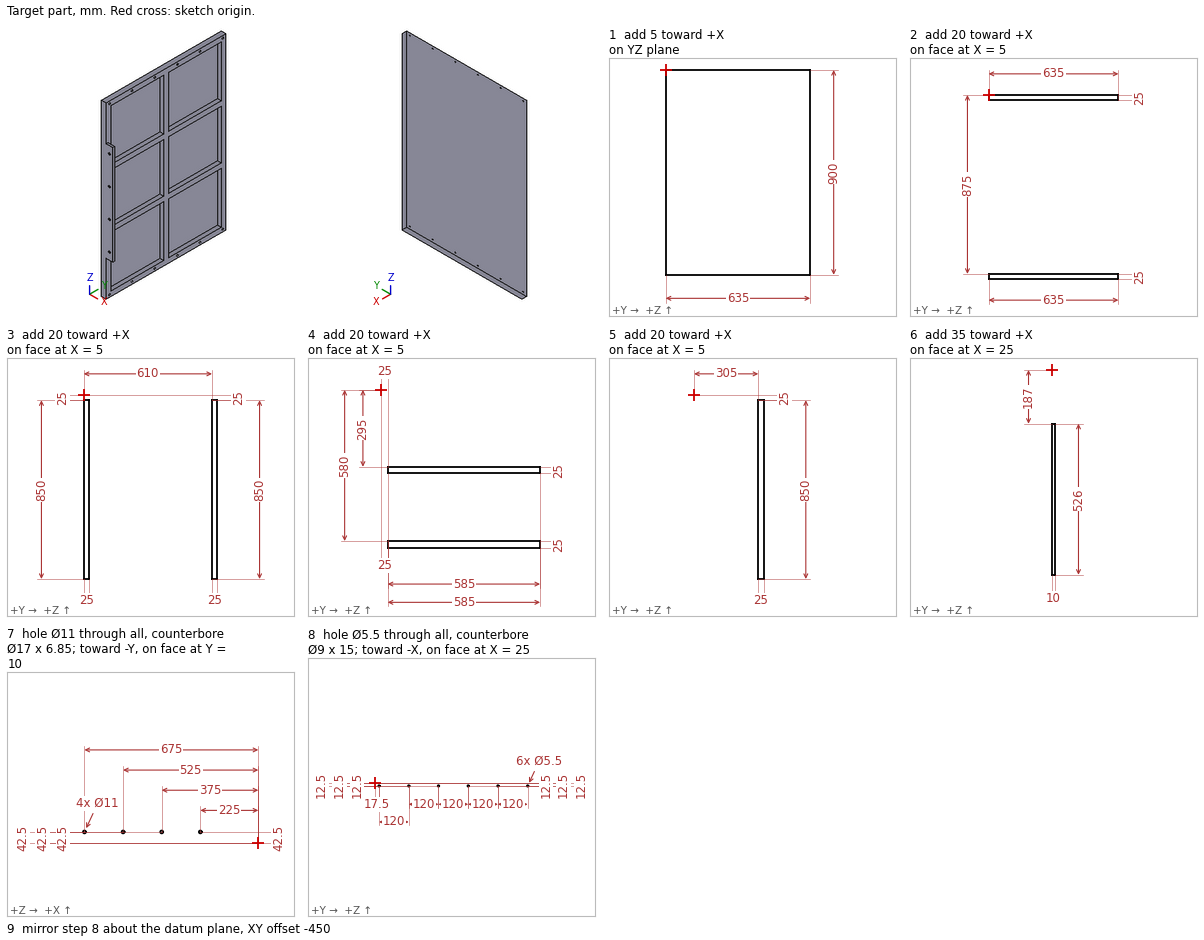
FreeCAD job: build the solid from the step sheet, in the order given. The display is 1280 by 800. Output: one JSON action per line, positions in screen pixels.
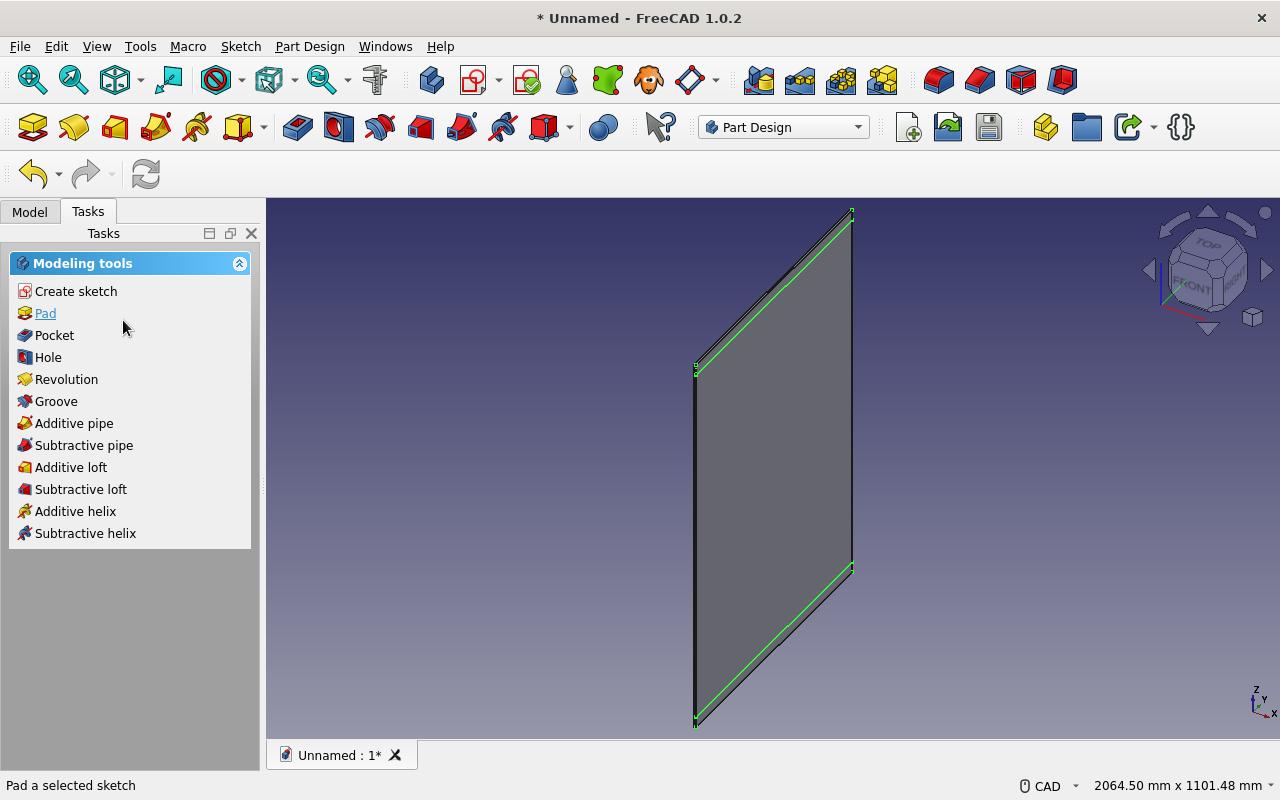
{"action": "left_click", "coordinate": [33, 128]}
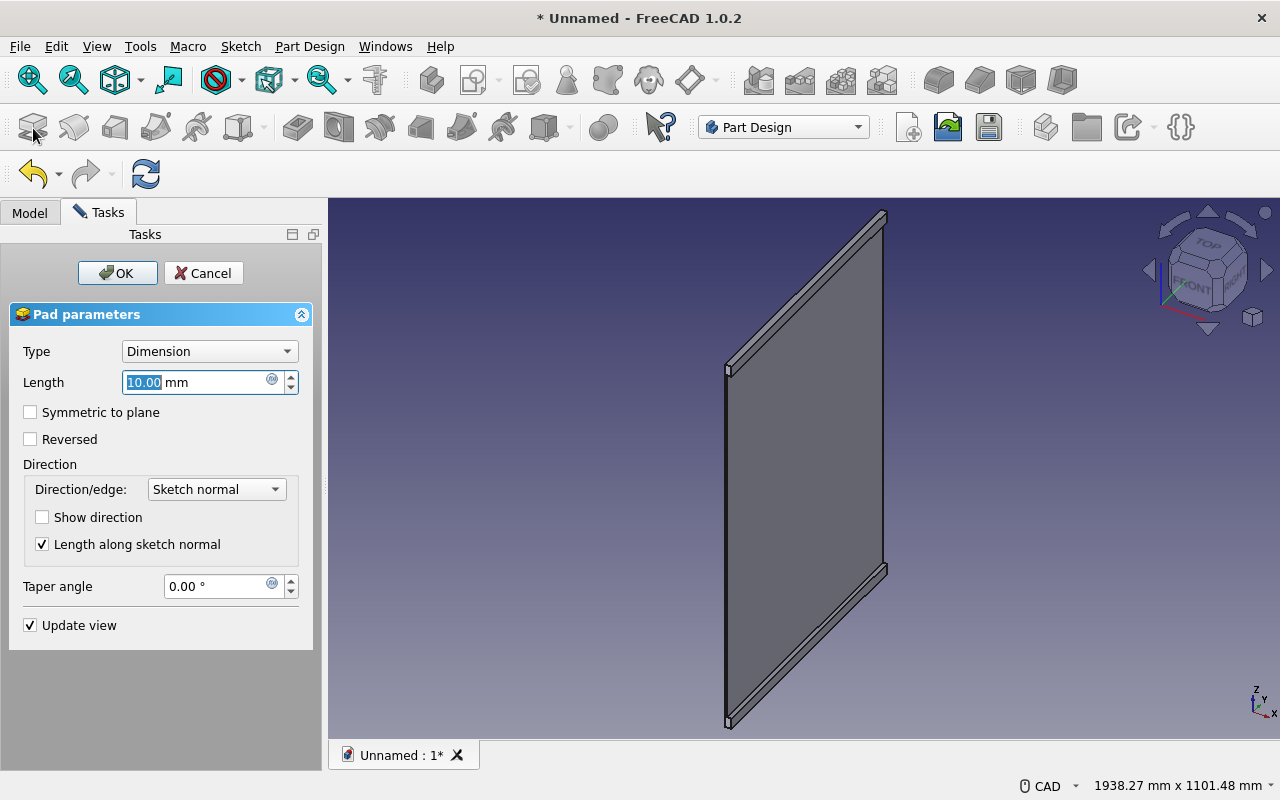
{"action": "type", "text": "20"}
{"action": "key", "text": "Tab"}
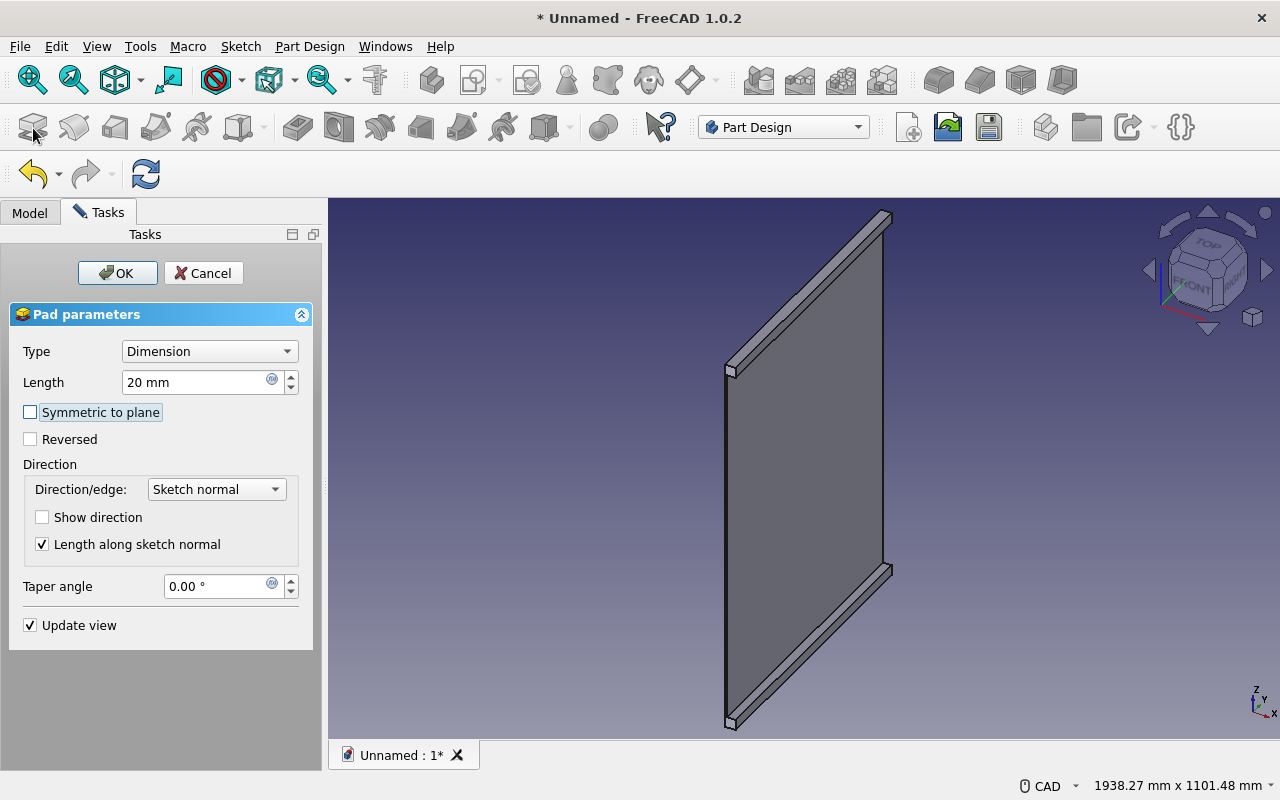
{"action": "left_click", "coordinate": [118, 273]}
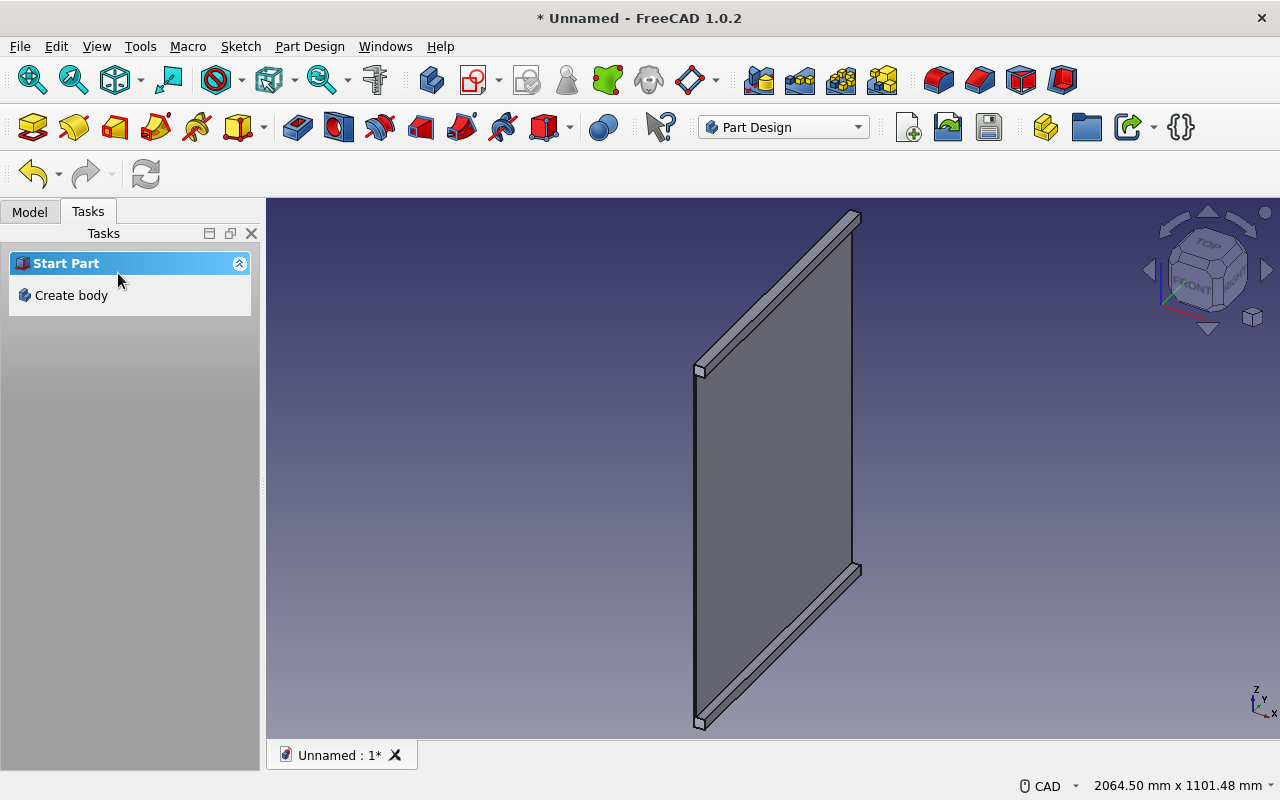
{"action": "left_click", "coordinate": [774, 468]}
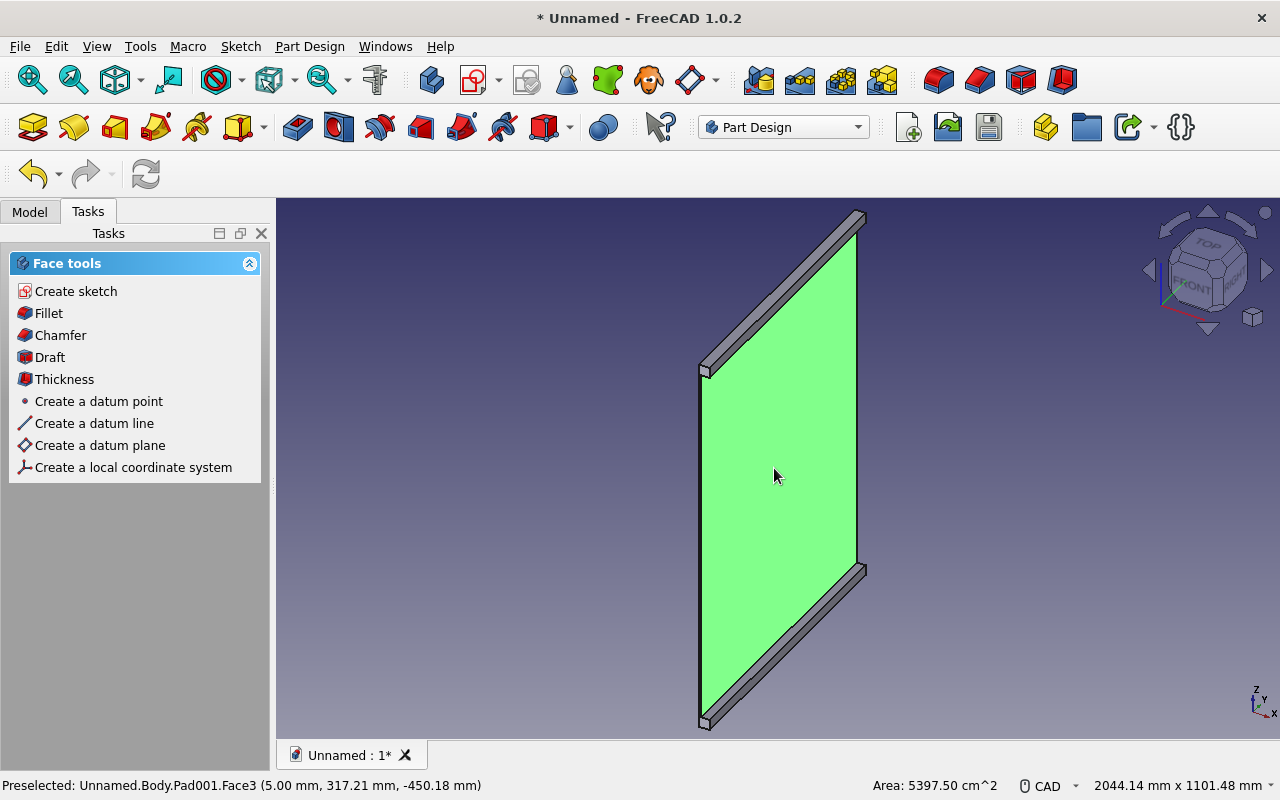
{"action": "left_click", "coordinate": [472, 80]}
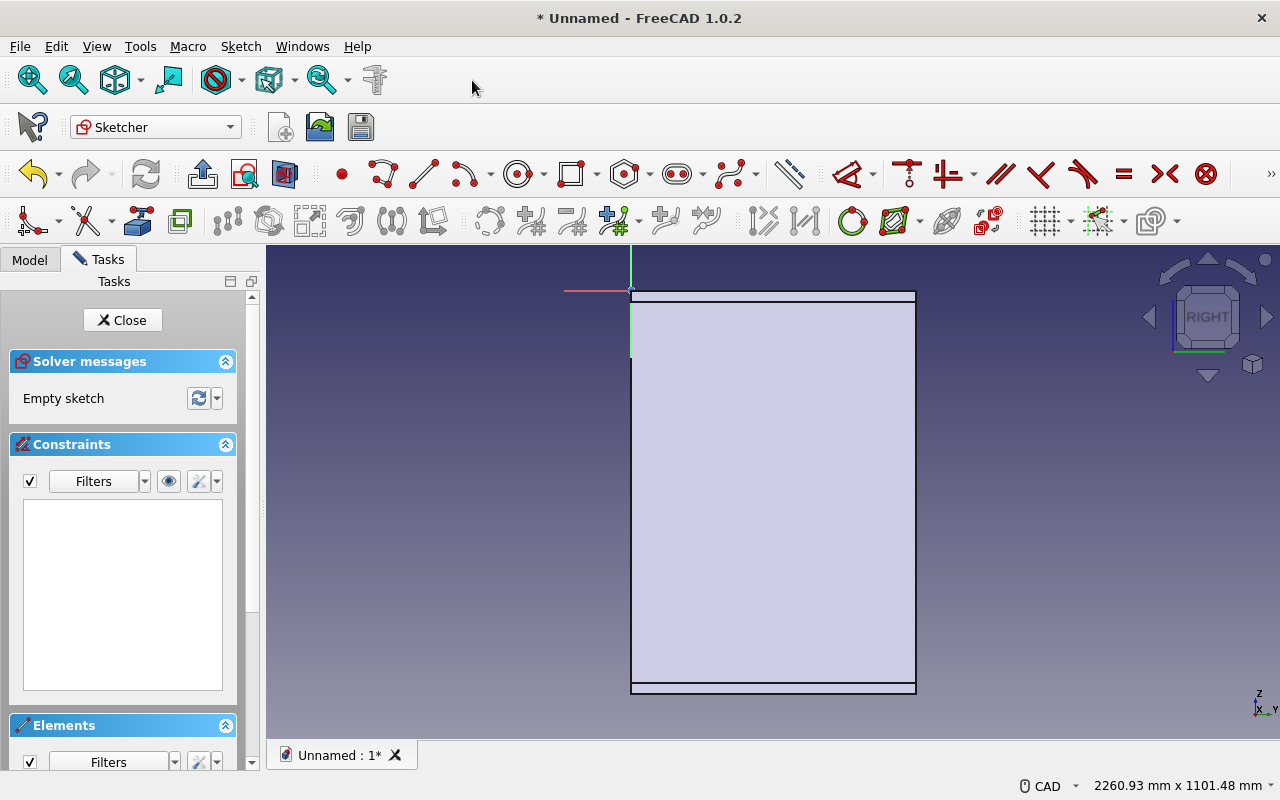
{"action": "scroll", "coordinate": [392, 515], "scroll_direction": "down", "scroll_amount": 1}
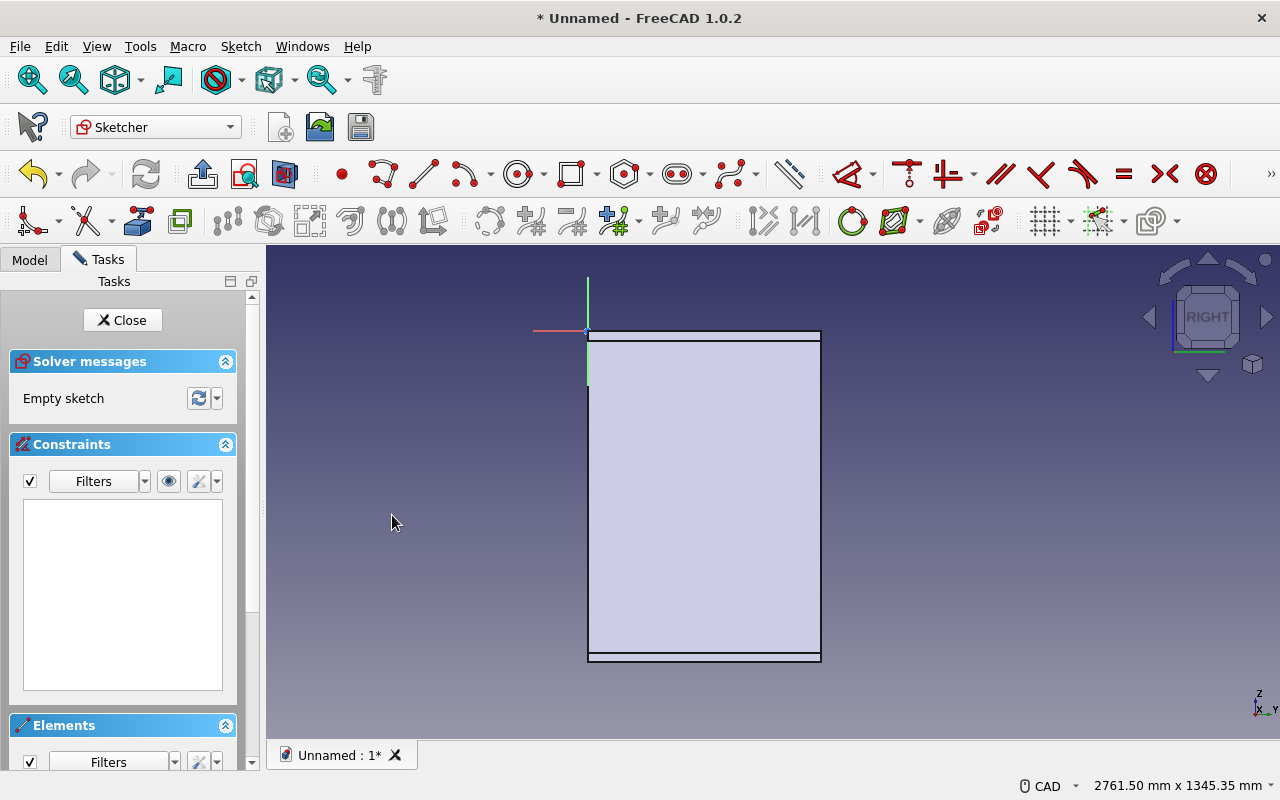
{"action": "left_click", "coordinate": [570, 174]}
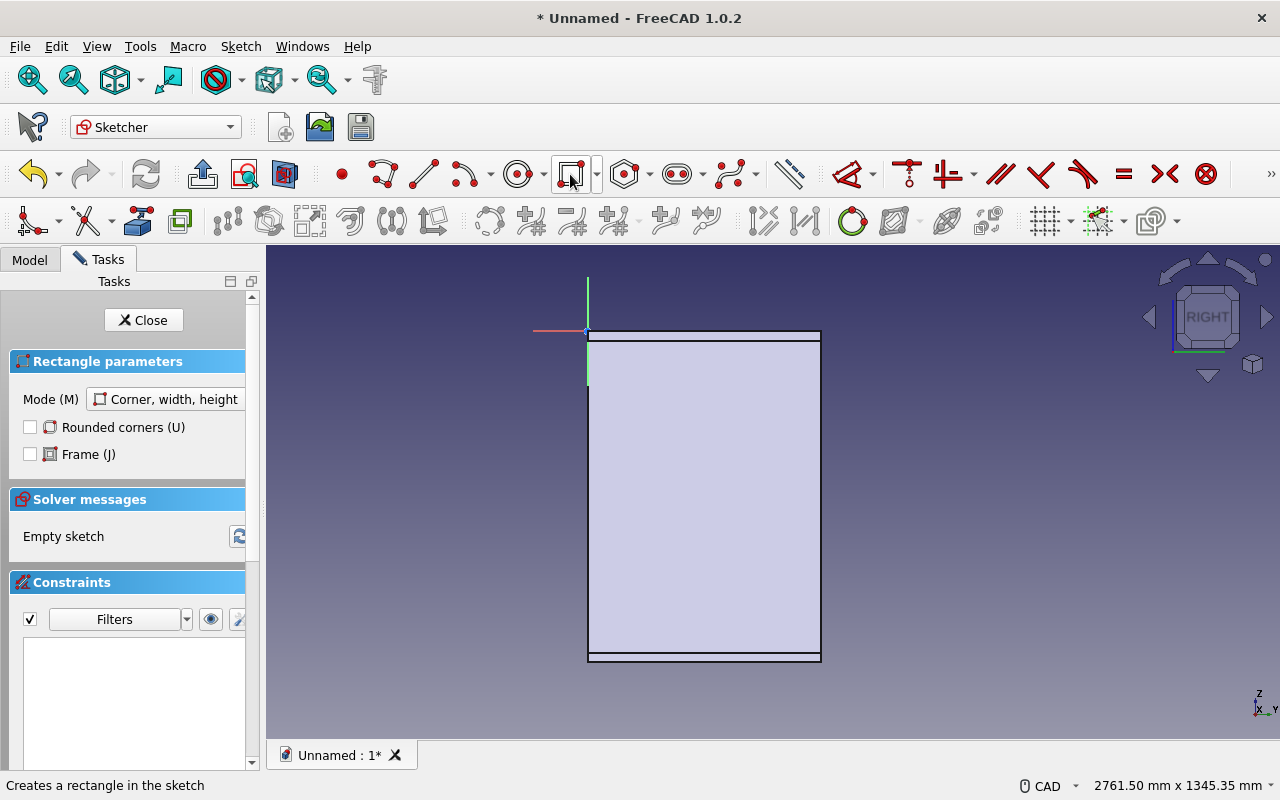
{"action": "scroll", "coordinate": [812, 341], "scroll_direction": "up", "scroll_amount": 3}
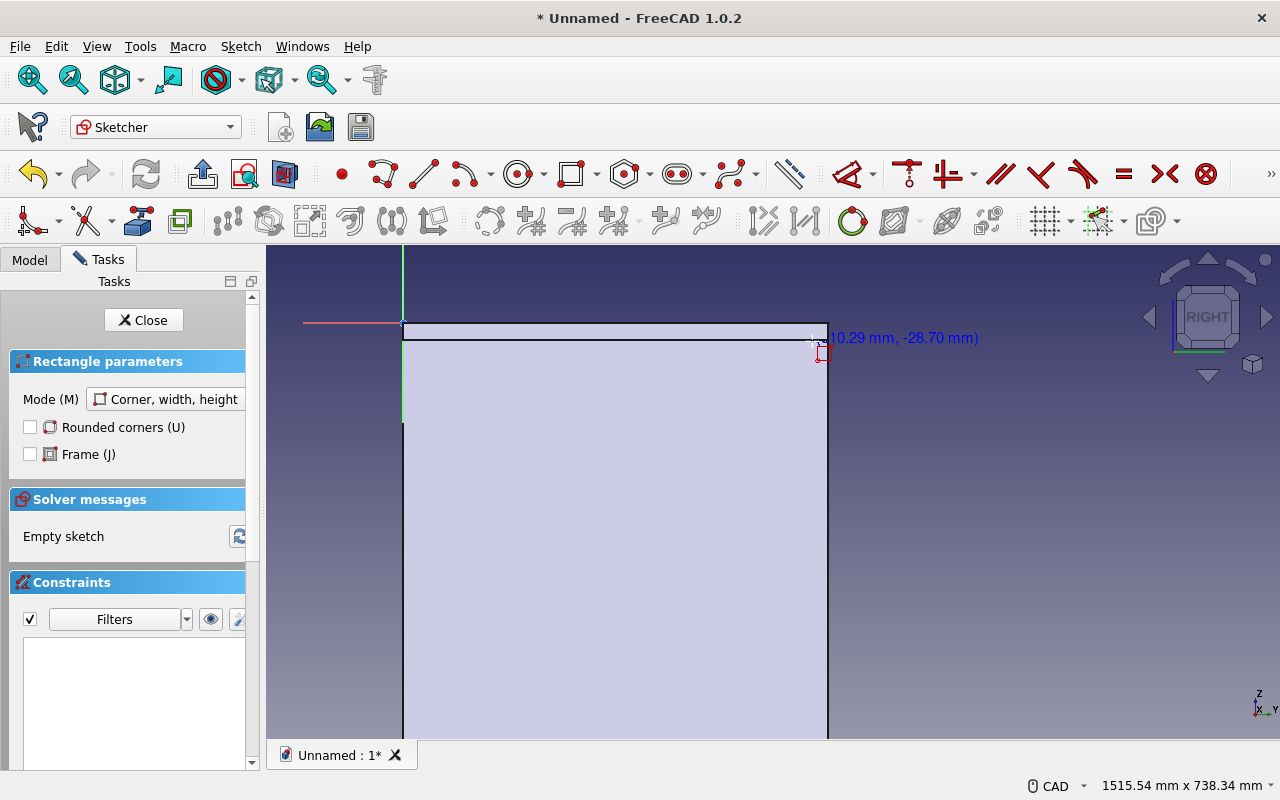
{"action": "left_click", "coordinate": [811, 340]}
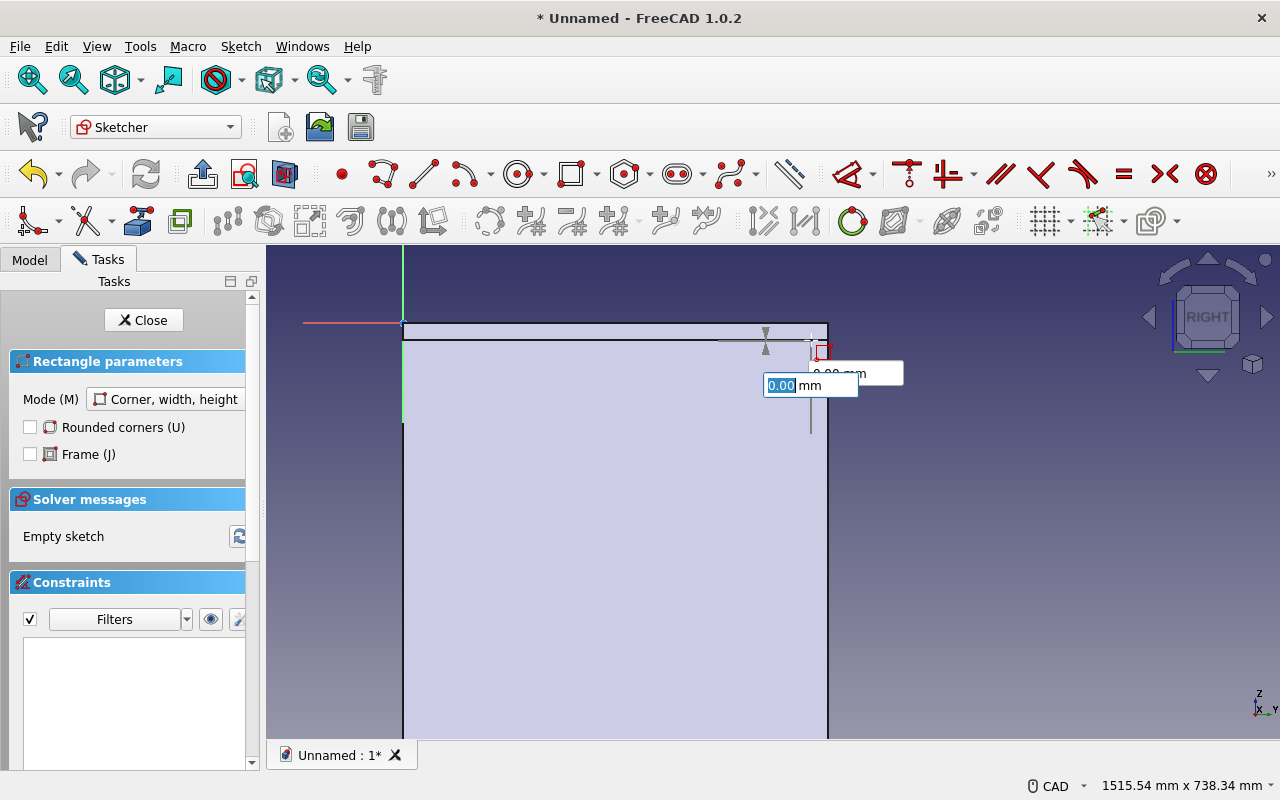
{"action": "scroll", "coordinate": [813, 341], "scroll_direction": "down", "scroll_amount": 3}